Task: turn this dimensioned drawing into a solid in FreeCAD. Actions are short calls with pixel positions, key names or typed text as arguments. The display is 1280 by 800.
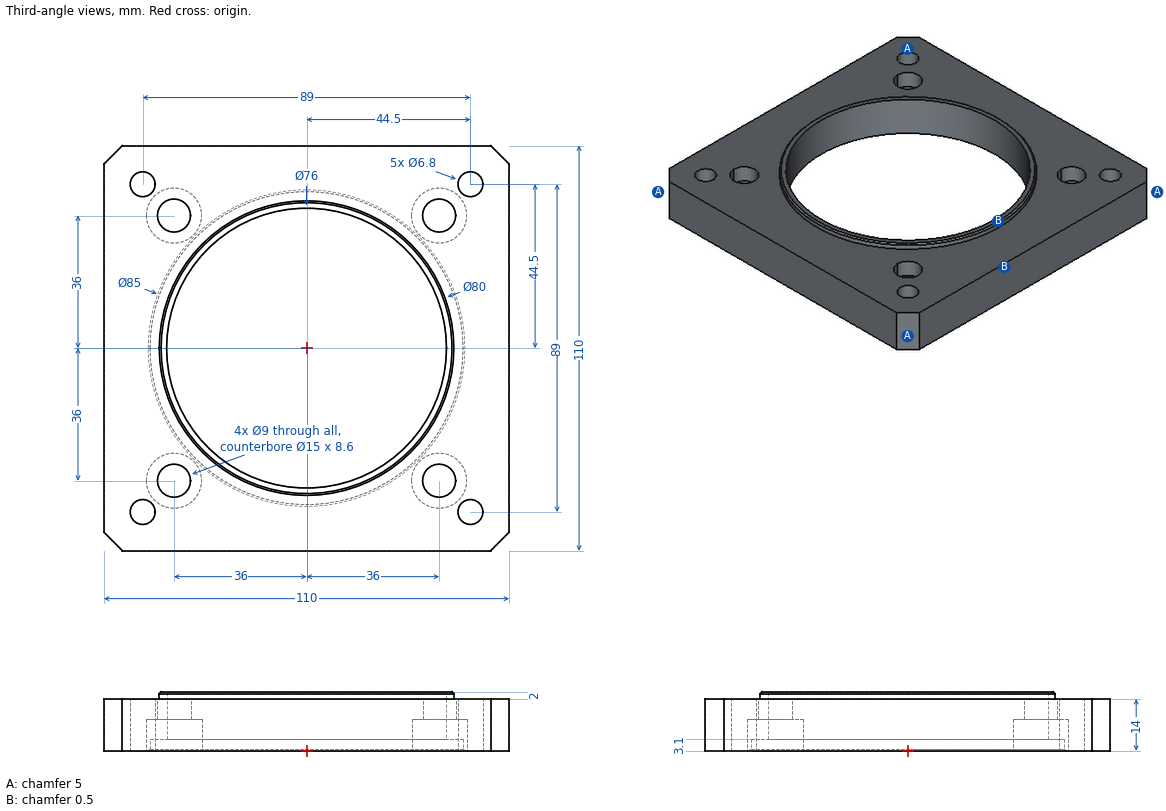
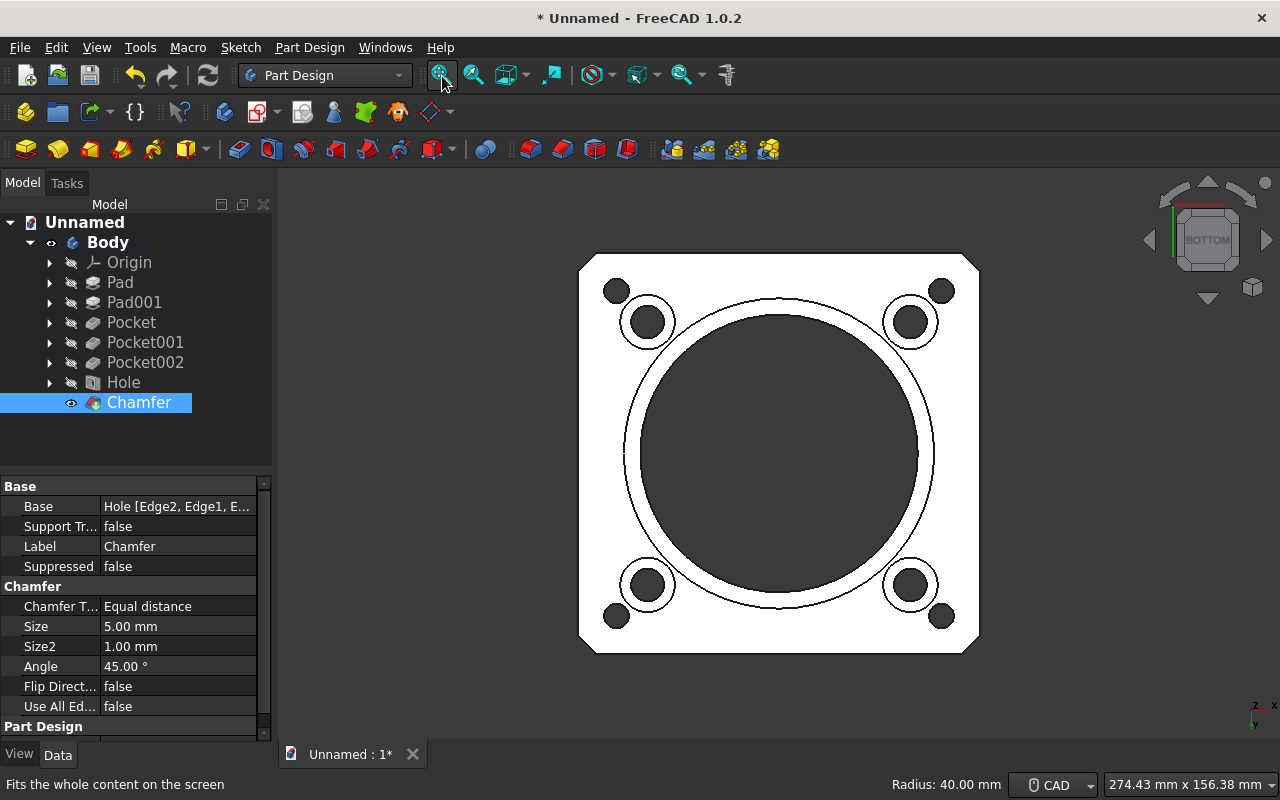
click(624, 452, ctrl)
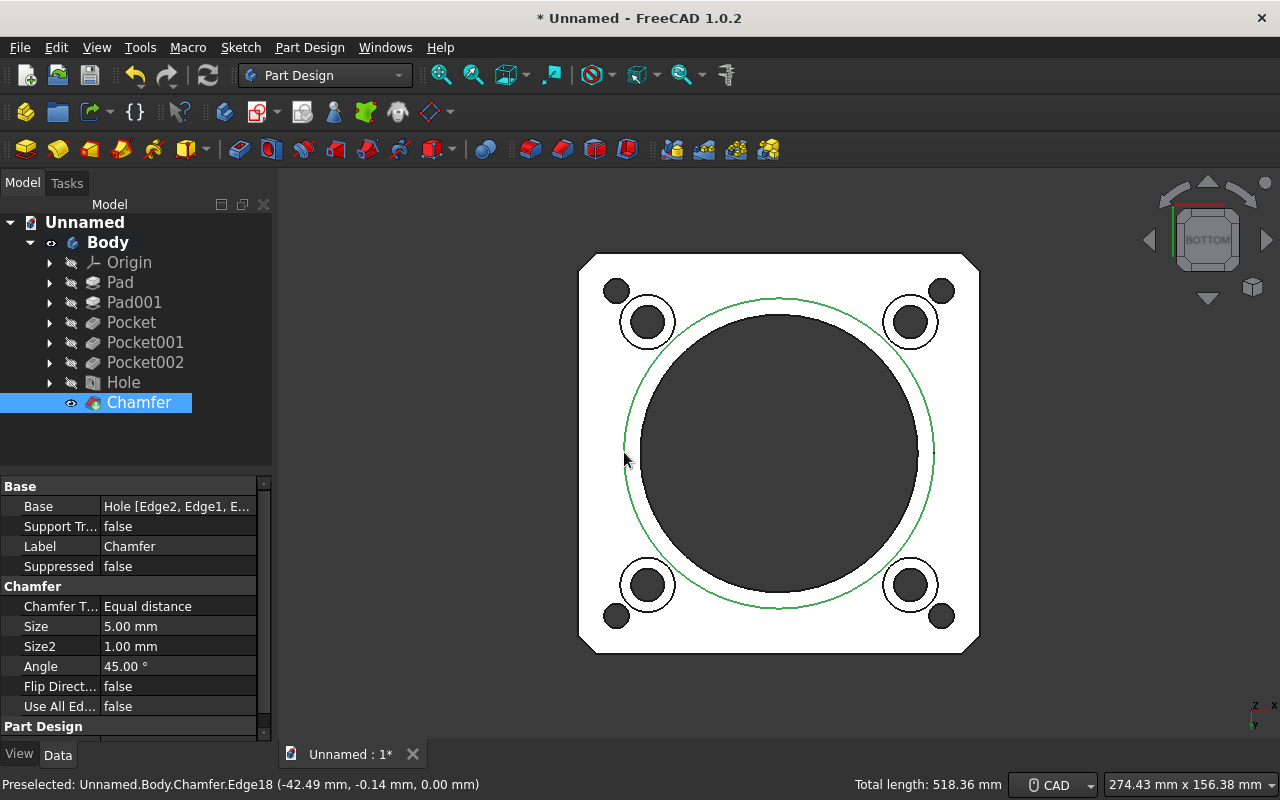
click(564, 150)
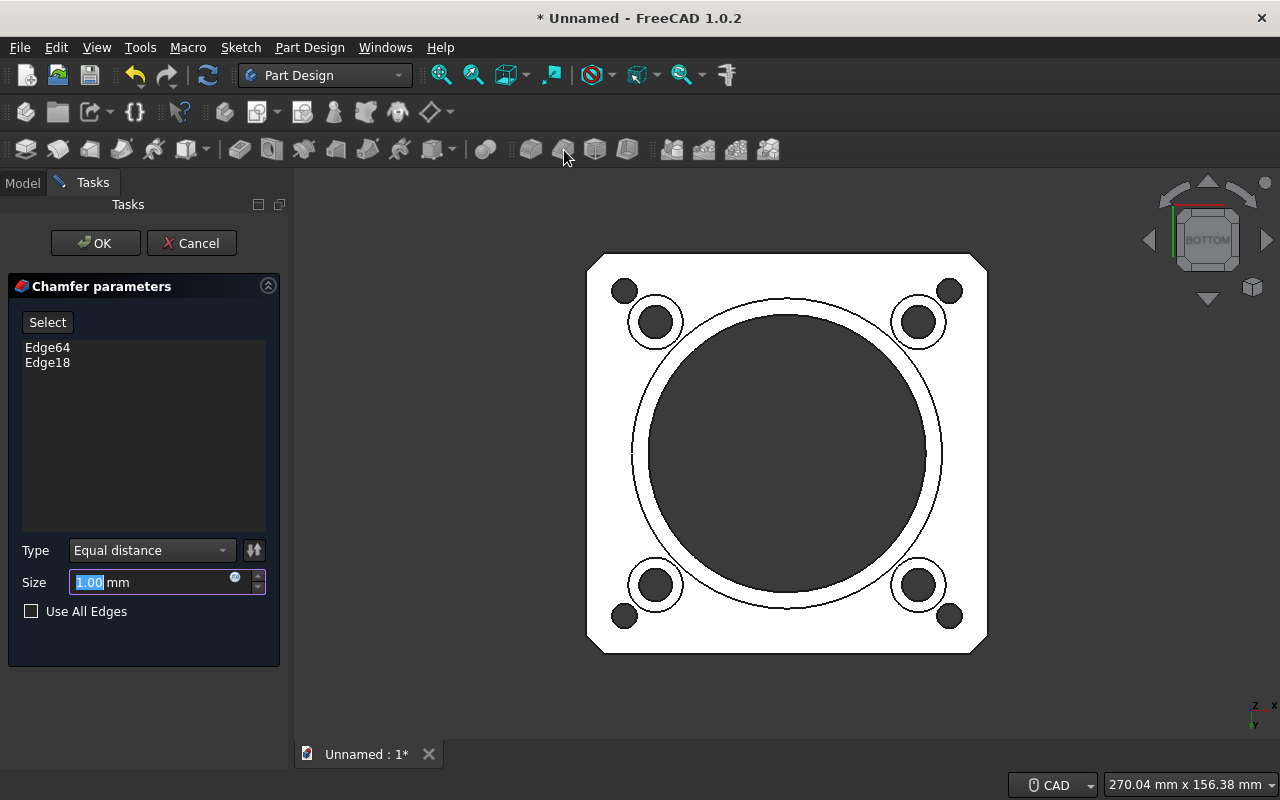
text(0.5)
key(Tab)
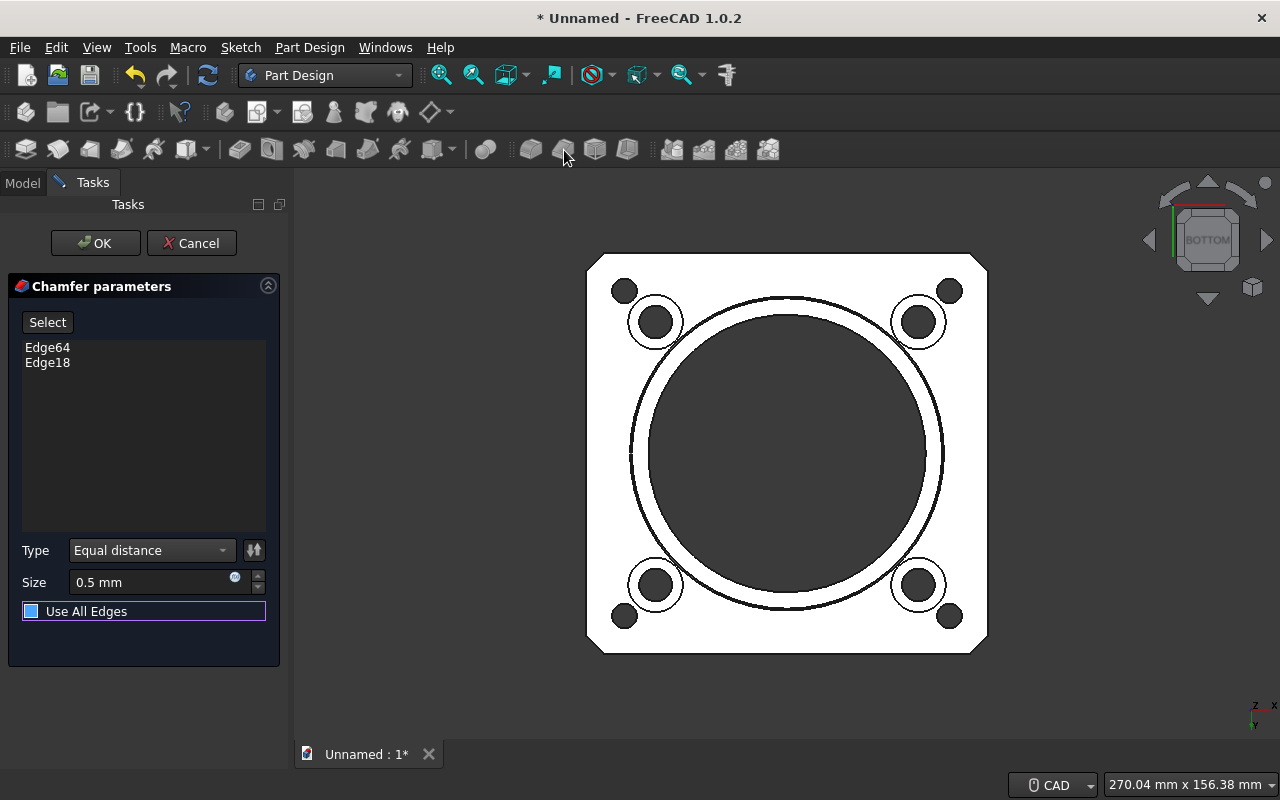
click(96, 243)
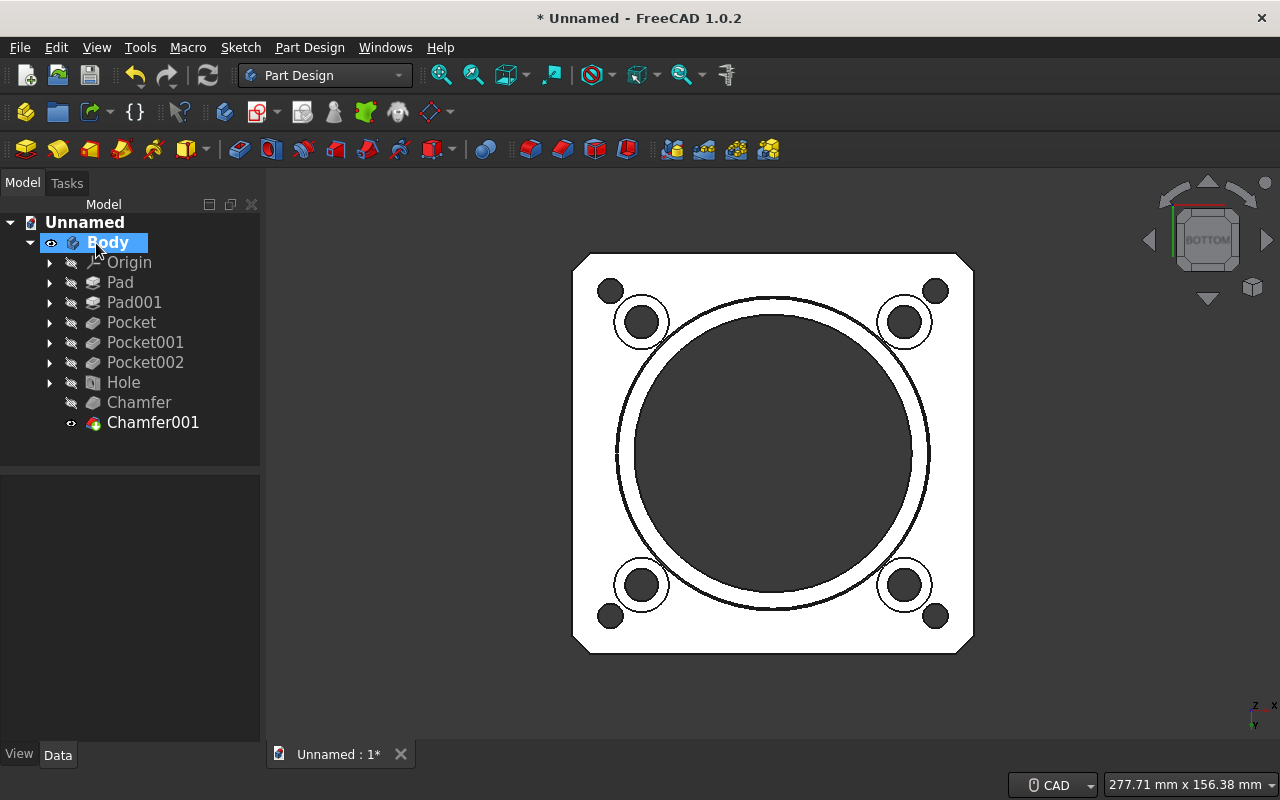
key(0)